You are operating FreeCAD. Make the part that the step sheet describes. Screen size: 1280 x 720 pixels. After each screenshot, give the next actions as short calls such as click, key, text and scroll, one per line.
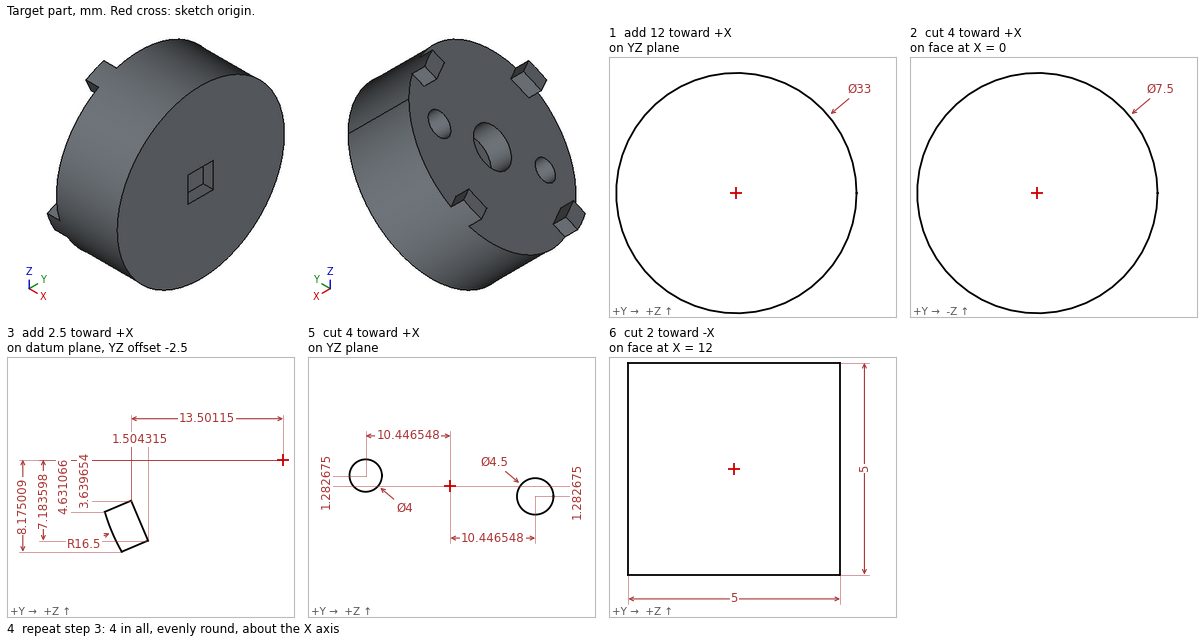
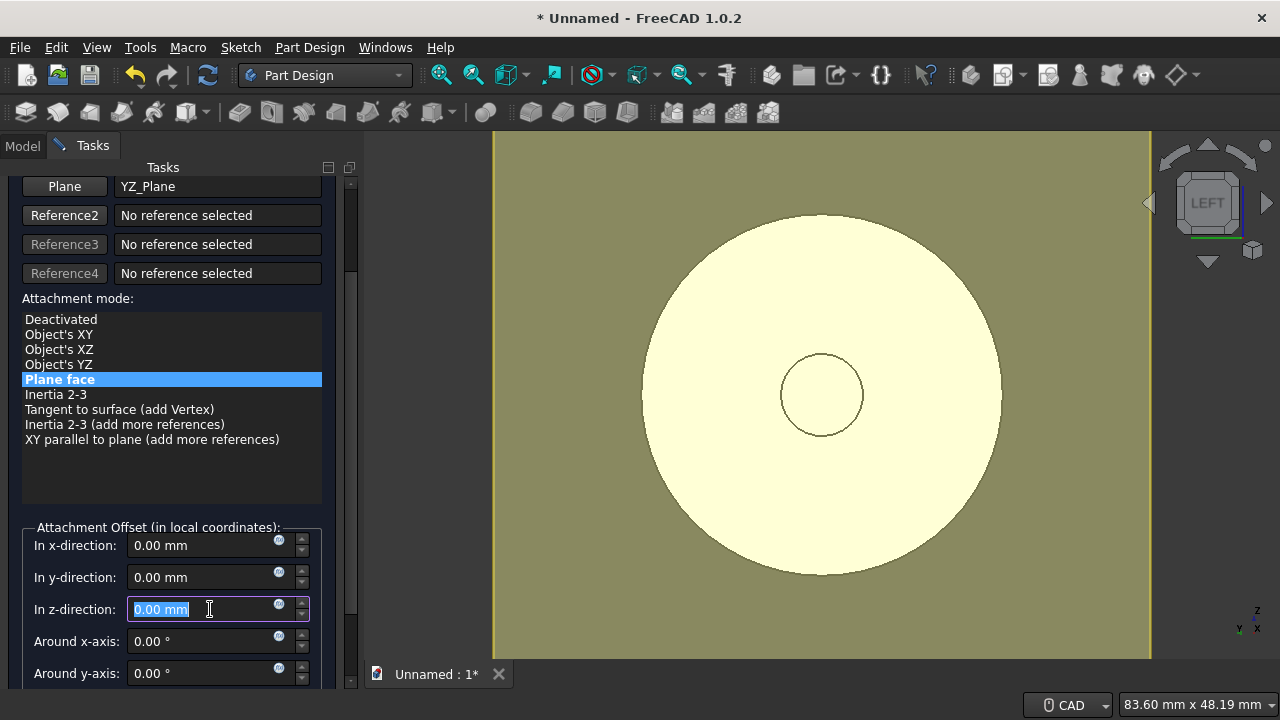
text(-2.5)
key(Tab)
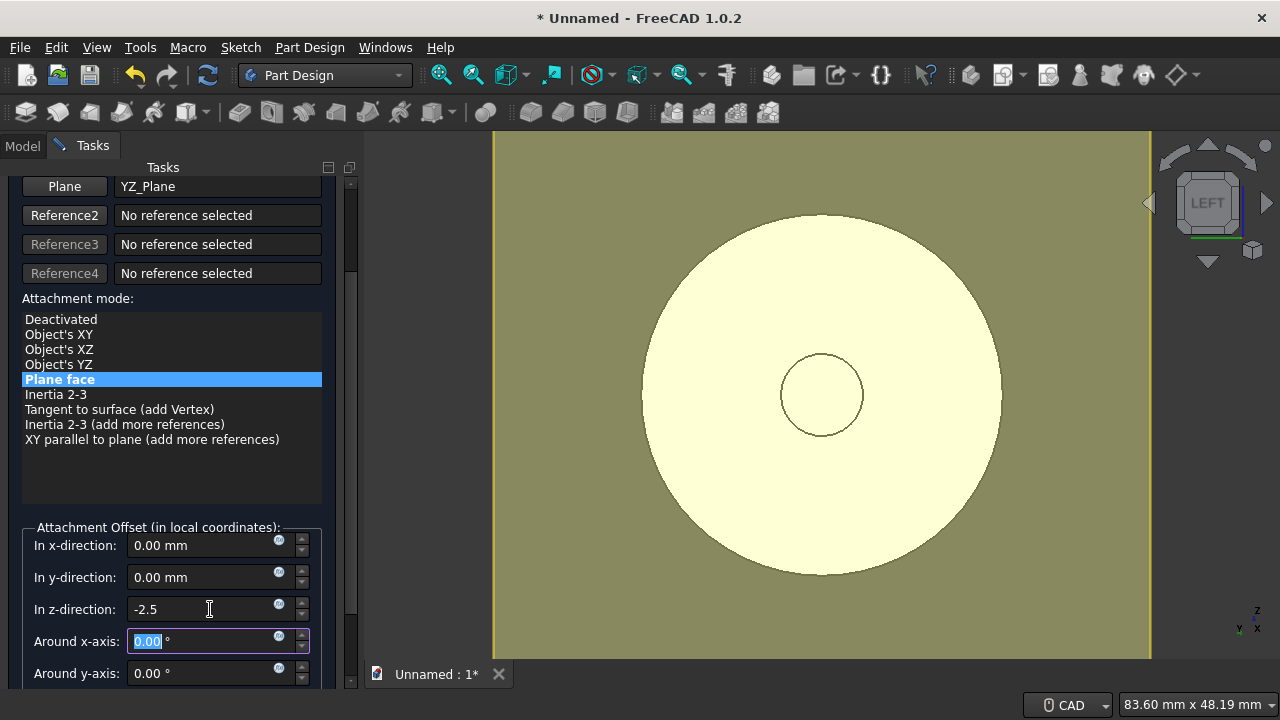
scroll(351, 432, up, 3)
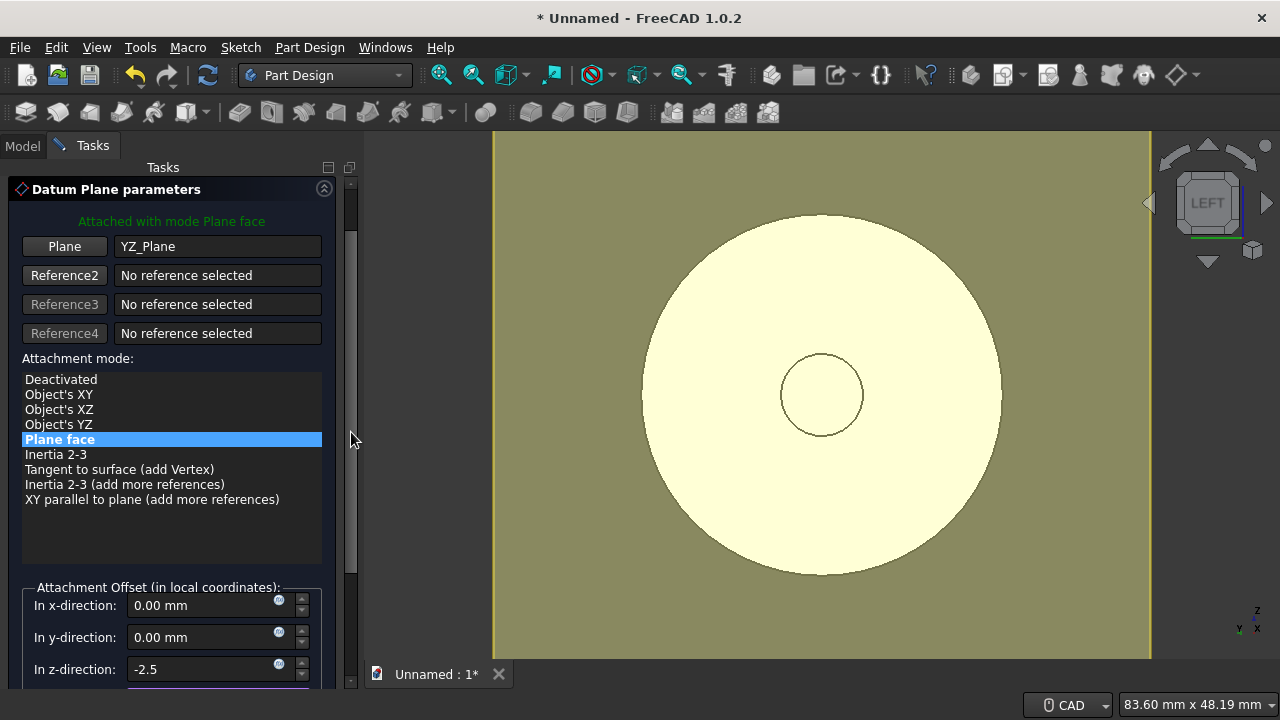
click(124, 206)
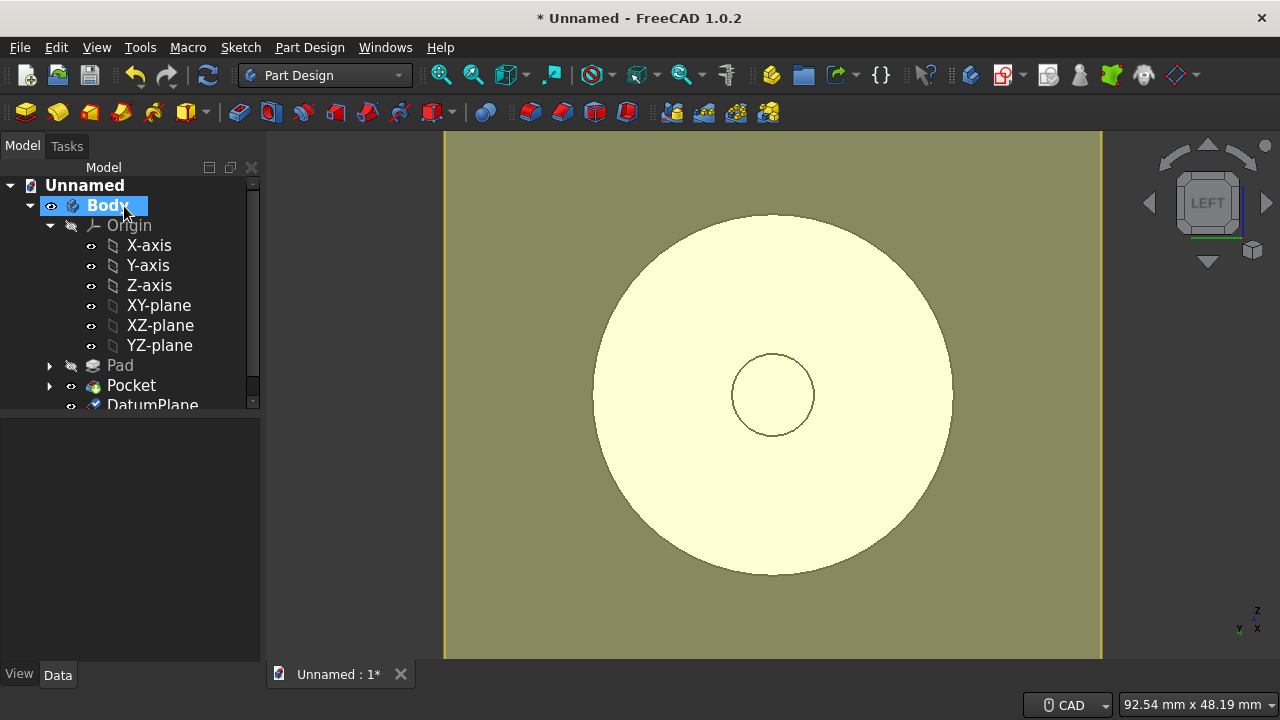
click(116, 406)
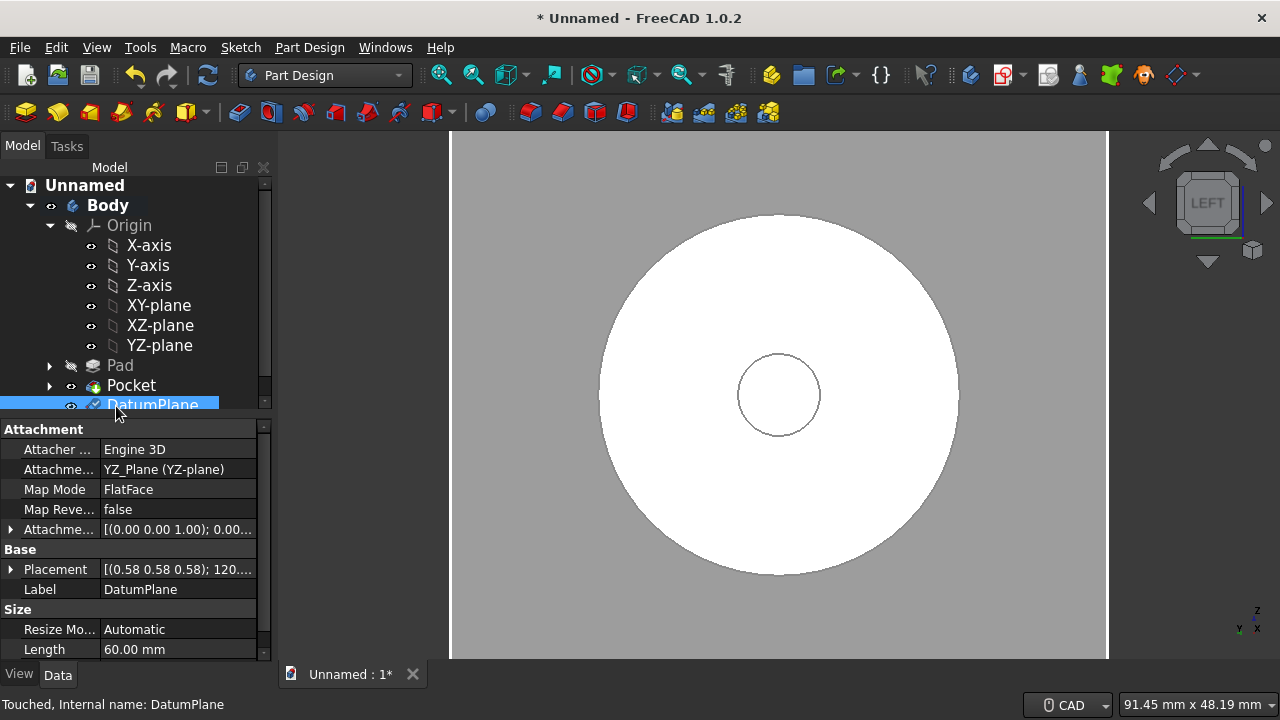
click(1004, 76)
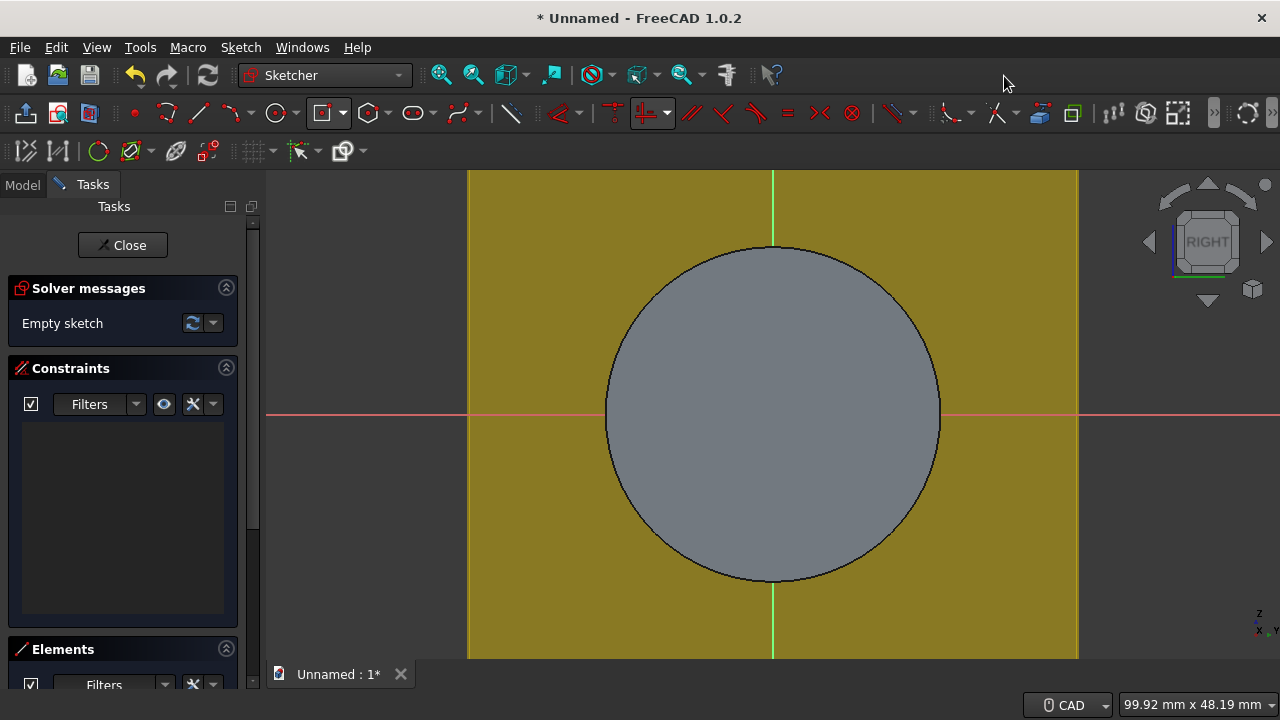
key(q)
key(s)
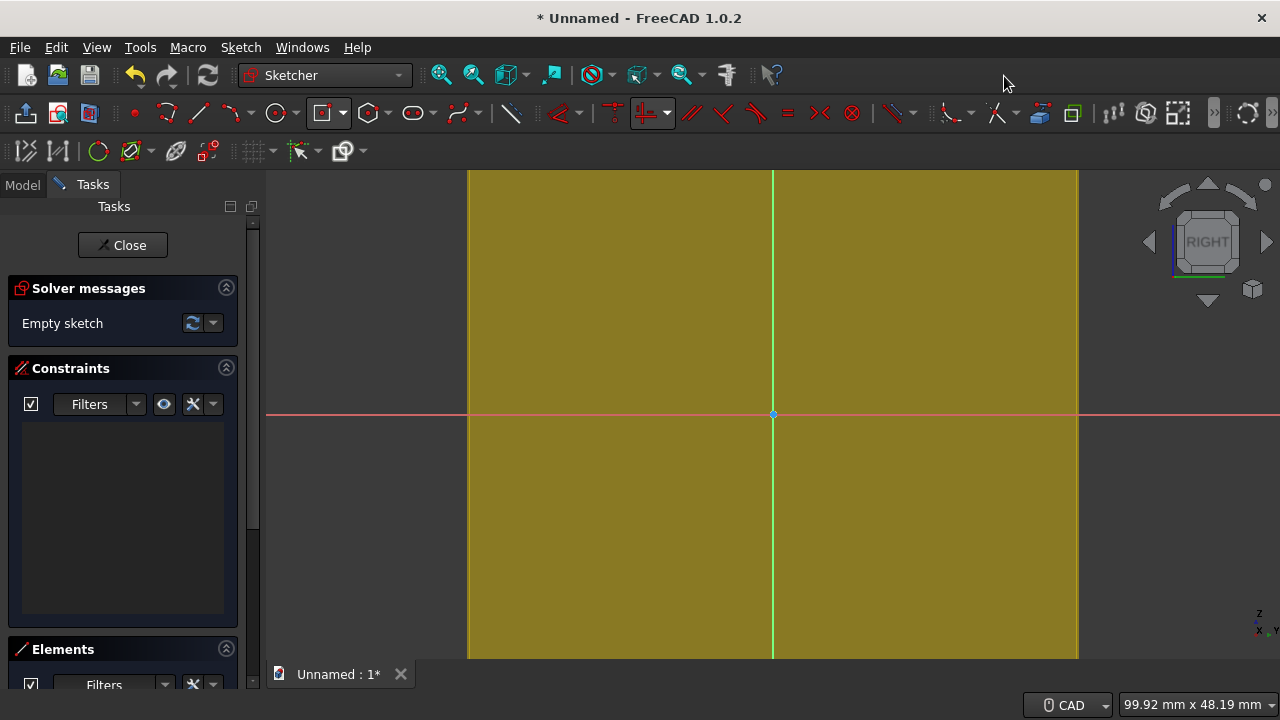
scroll(617, 486, up, 9)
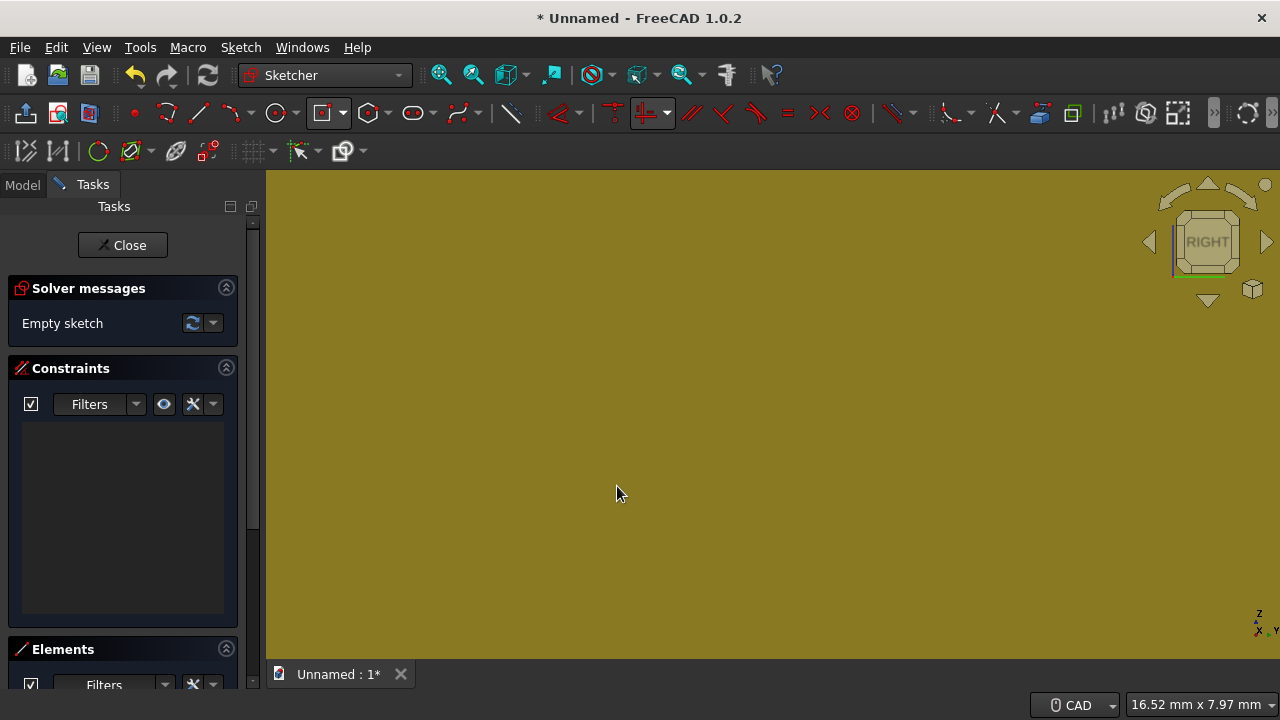
key(g)
key(m)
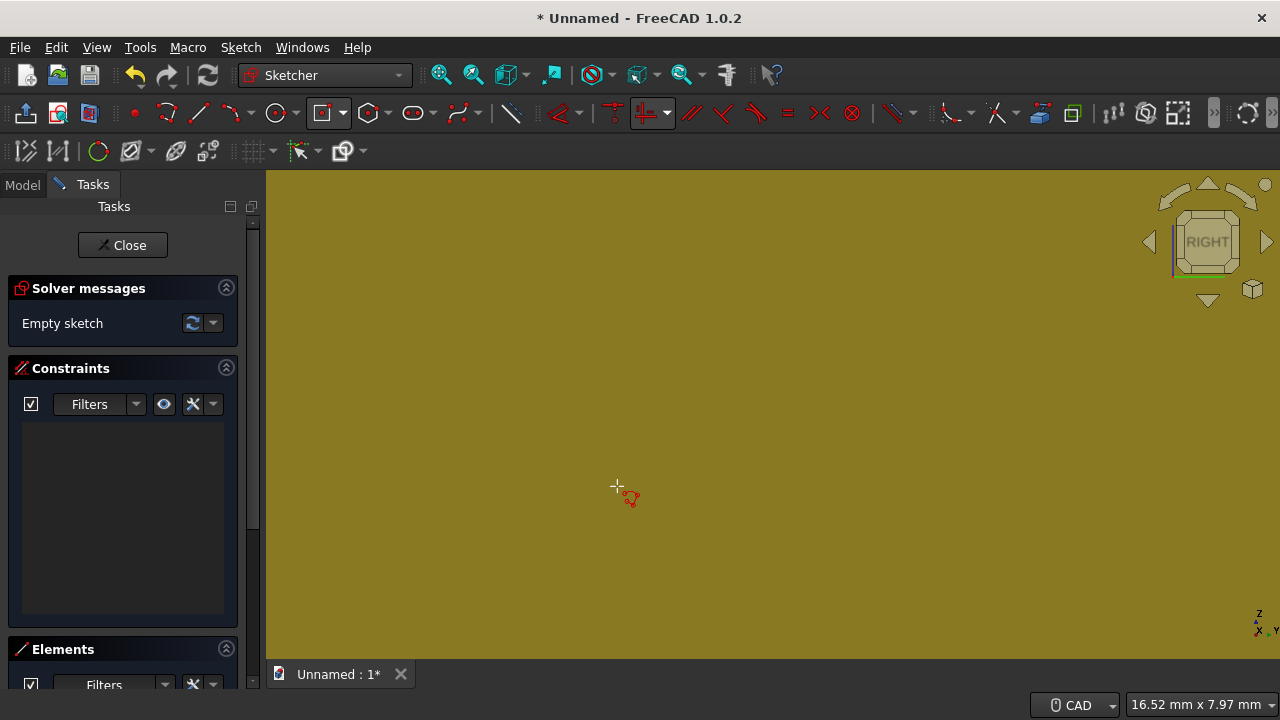
click(587, 334)
click(730, 274)
click(822, 491)
click(679, 552)
right_click(679, 552)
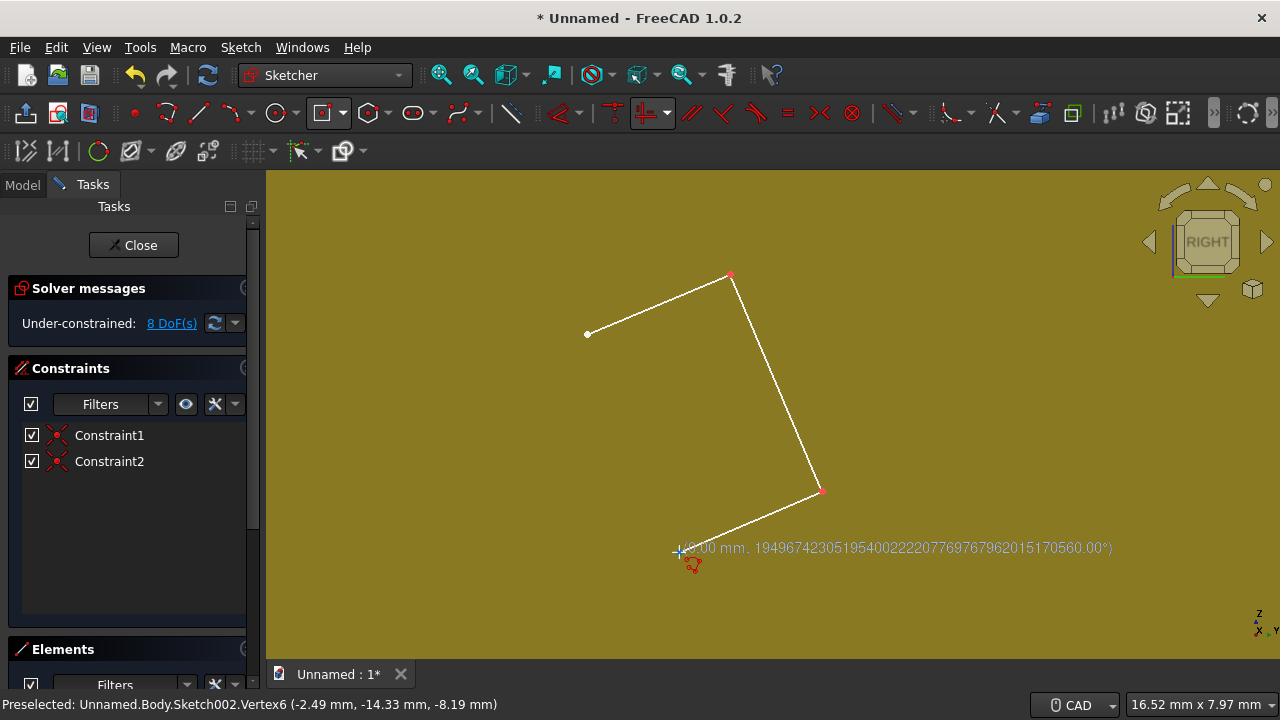
click(232, 114)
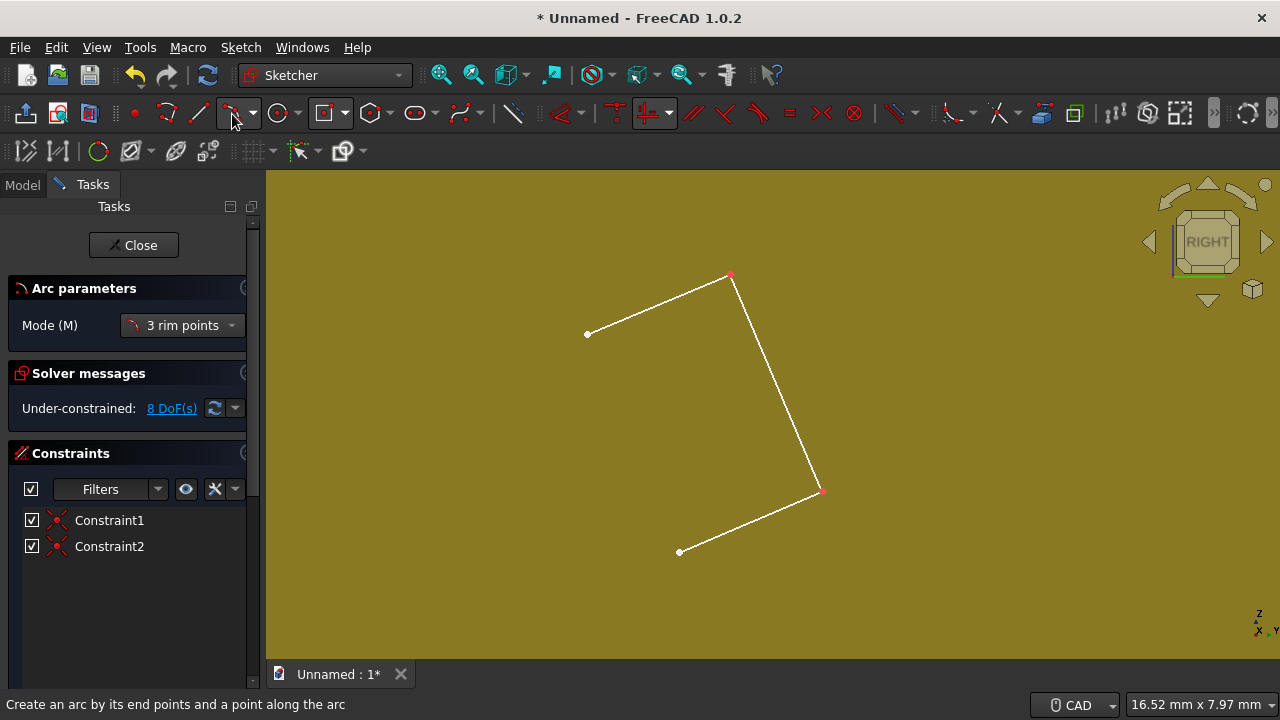
click(679, 553)
click(587, 335)